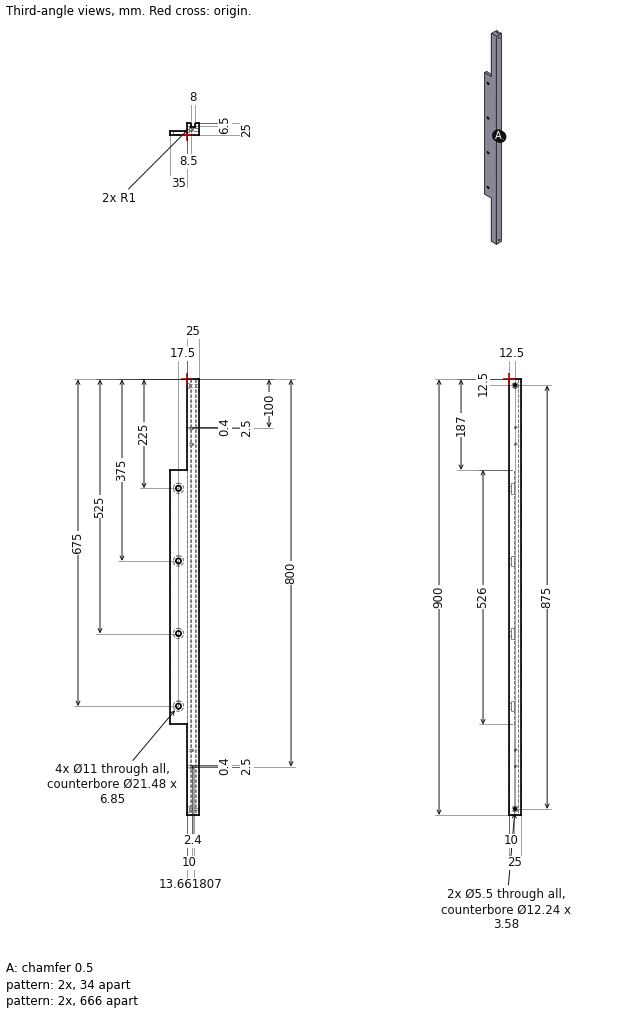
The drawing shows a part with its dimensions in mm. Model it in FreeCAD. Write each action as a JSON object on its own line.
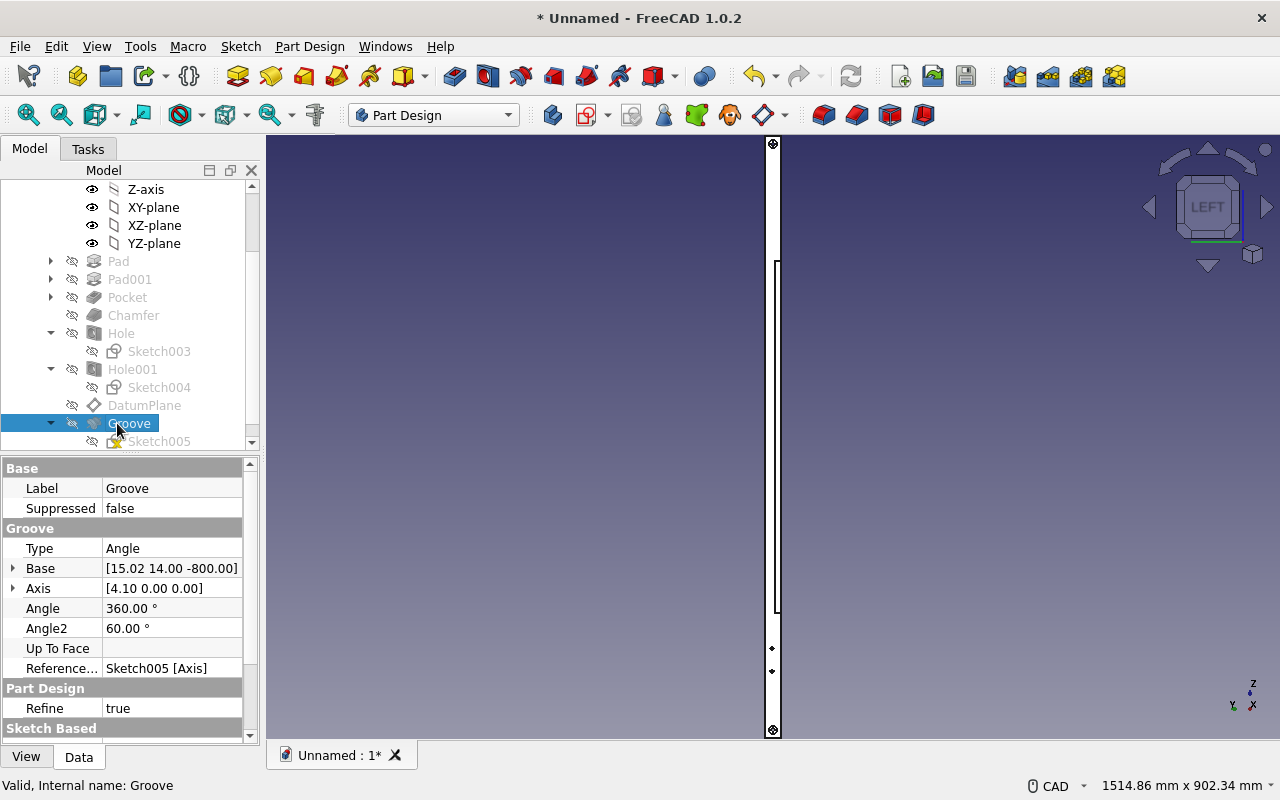
{"action": "left_click", "coordinate": [1048, 76]}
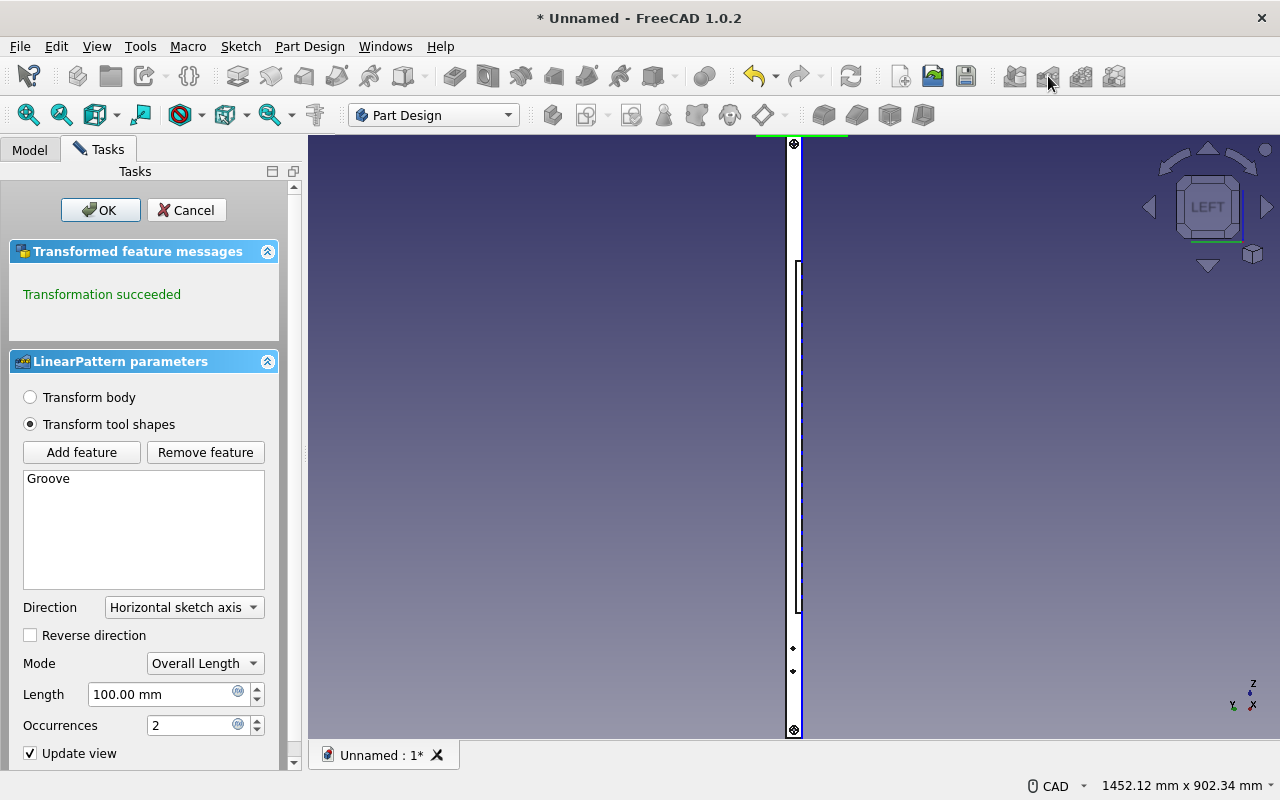
{"action": "left_click", "coordinate": [185, 608]}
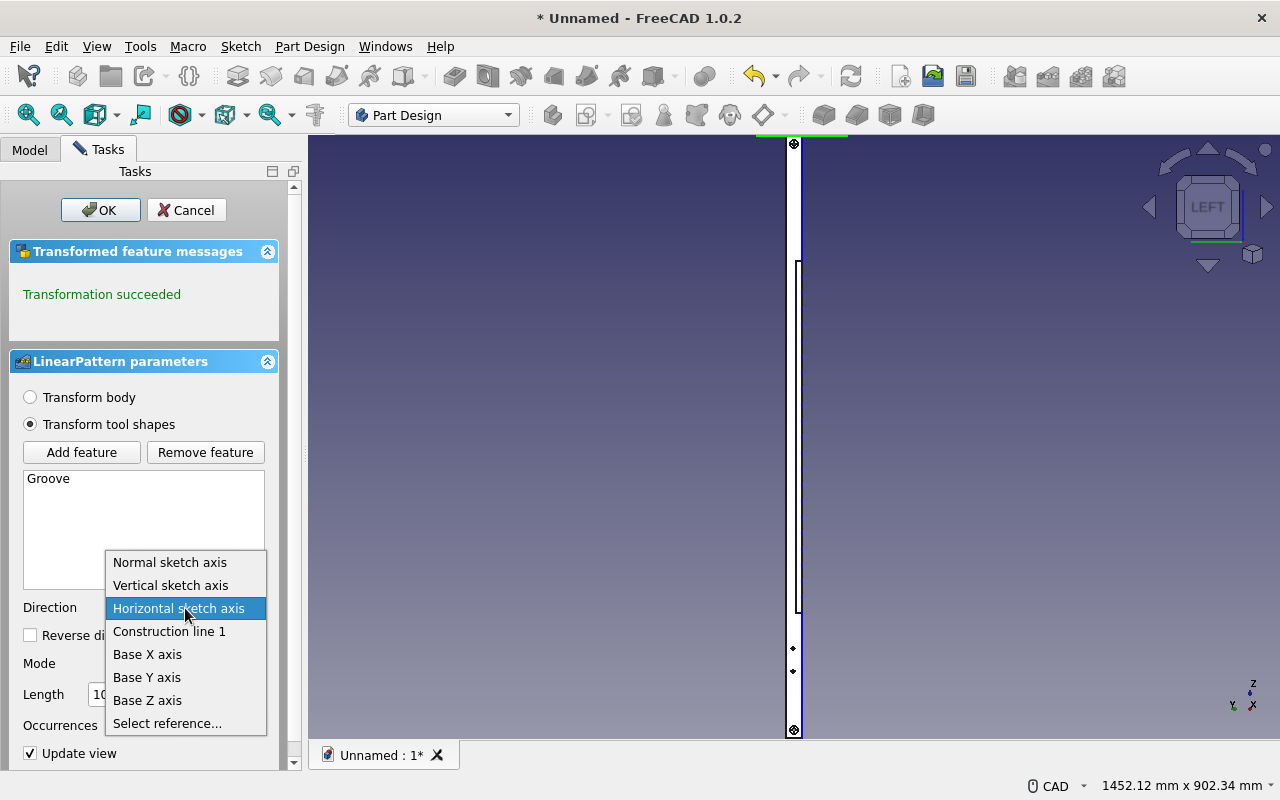
{"action": "left_click", "coordinate": [184, 700]}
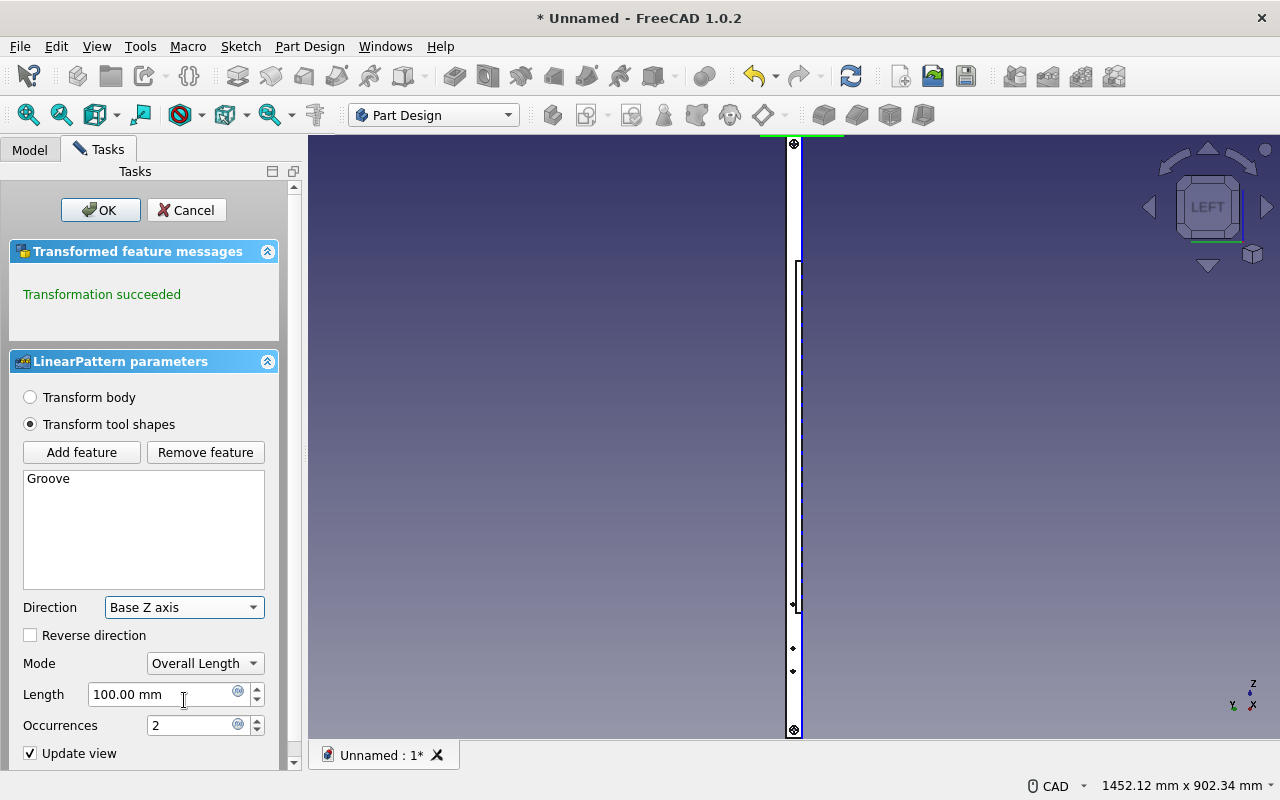
{"action": "left_click", "coordinate": [206, 664]}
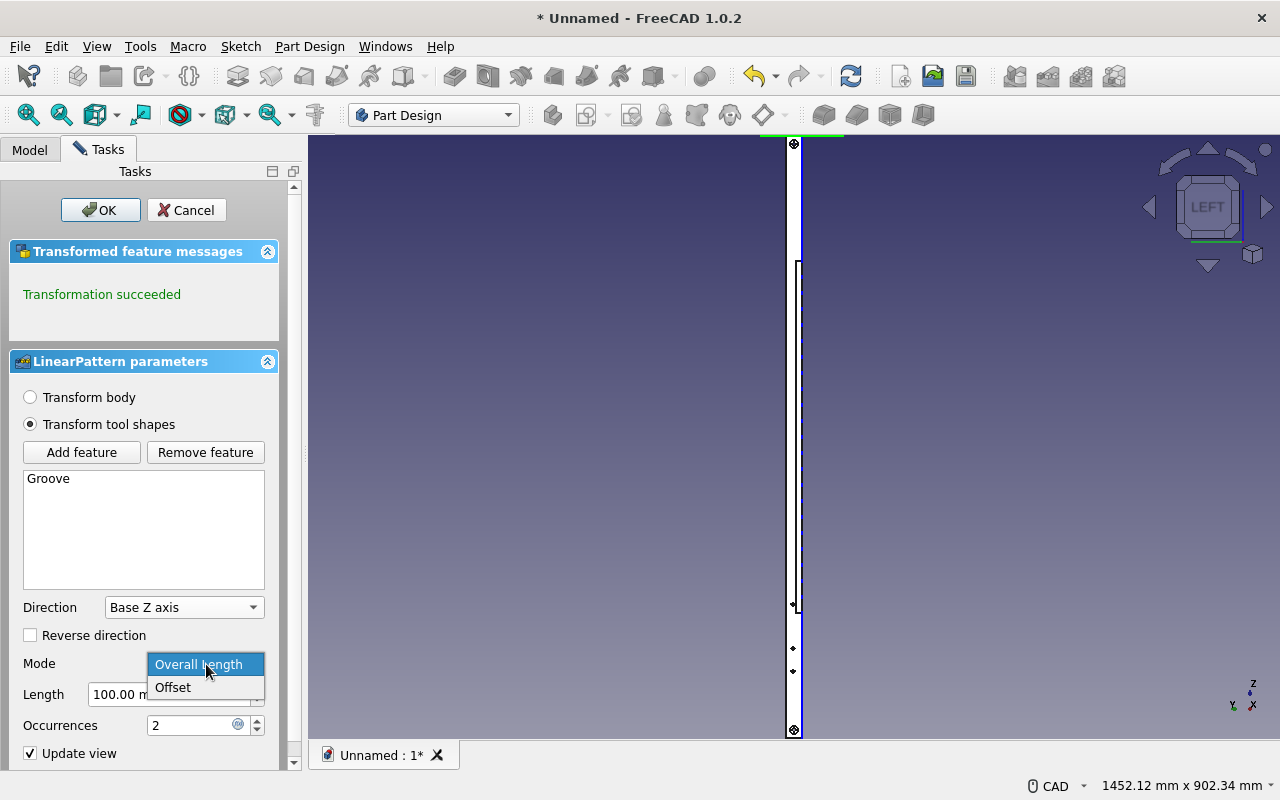
{"action": "left_click", "coordinate": [204, 688]}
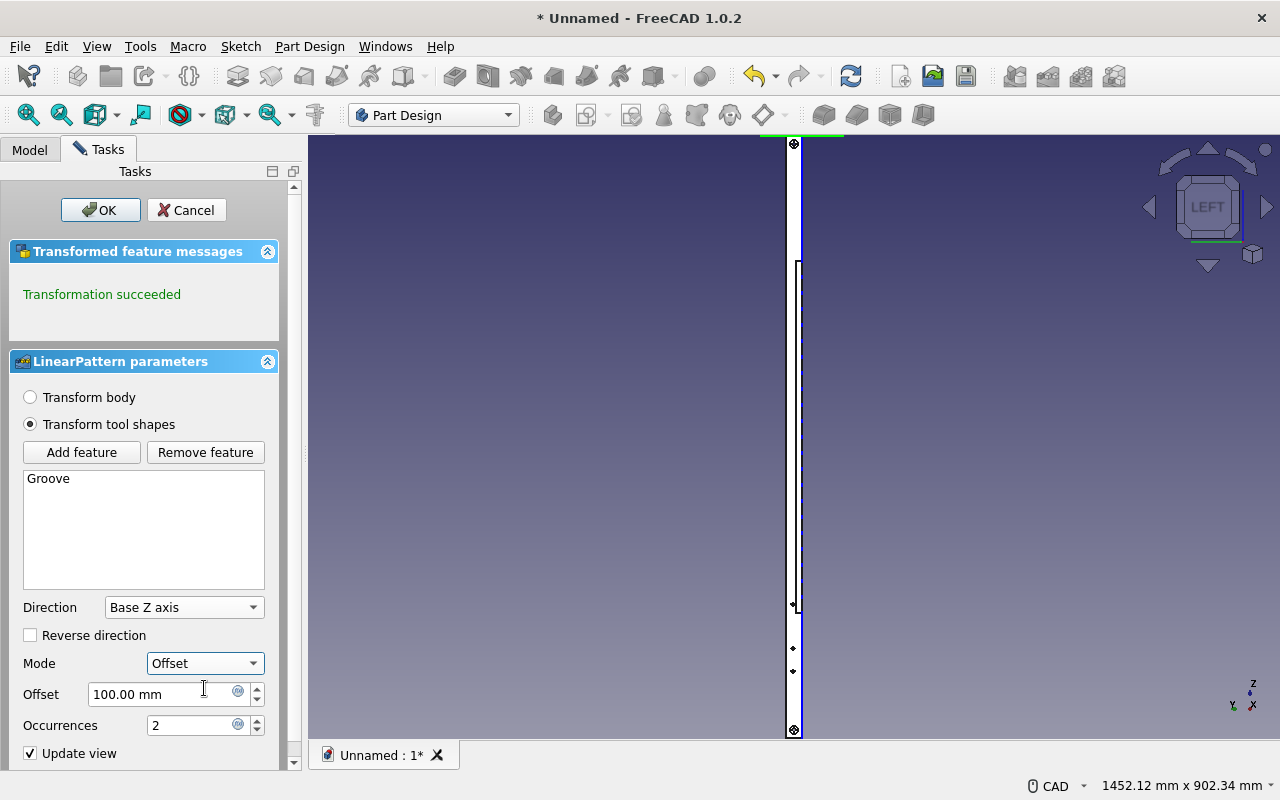
{"action": "triple_click", "coordinate": [170, 694]}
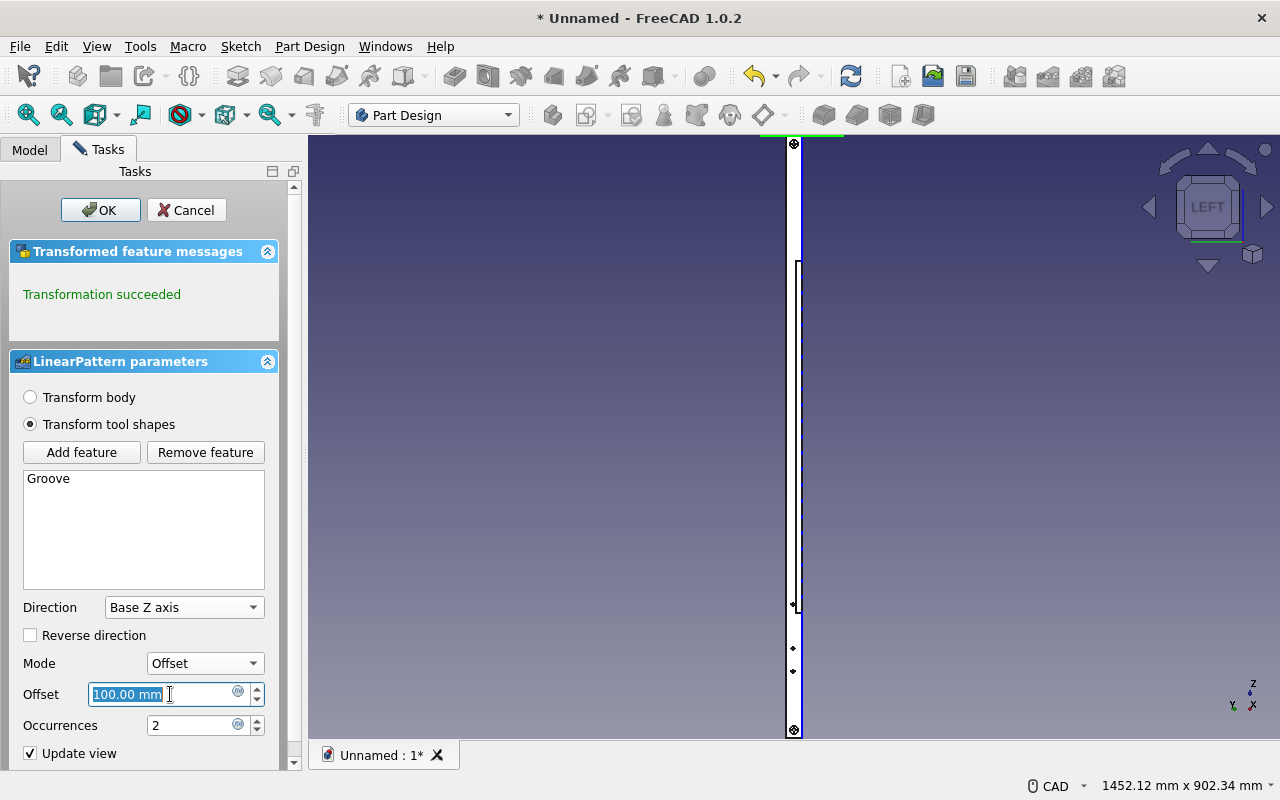
{"action": "type", "text": "666"}
{"action": "key", "text": "Tab"}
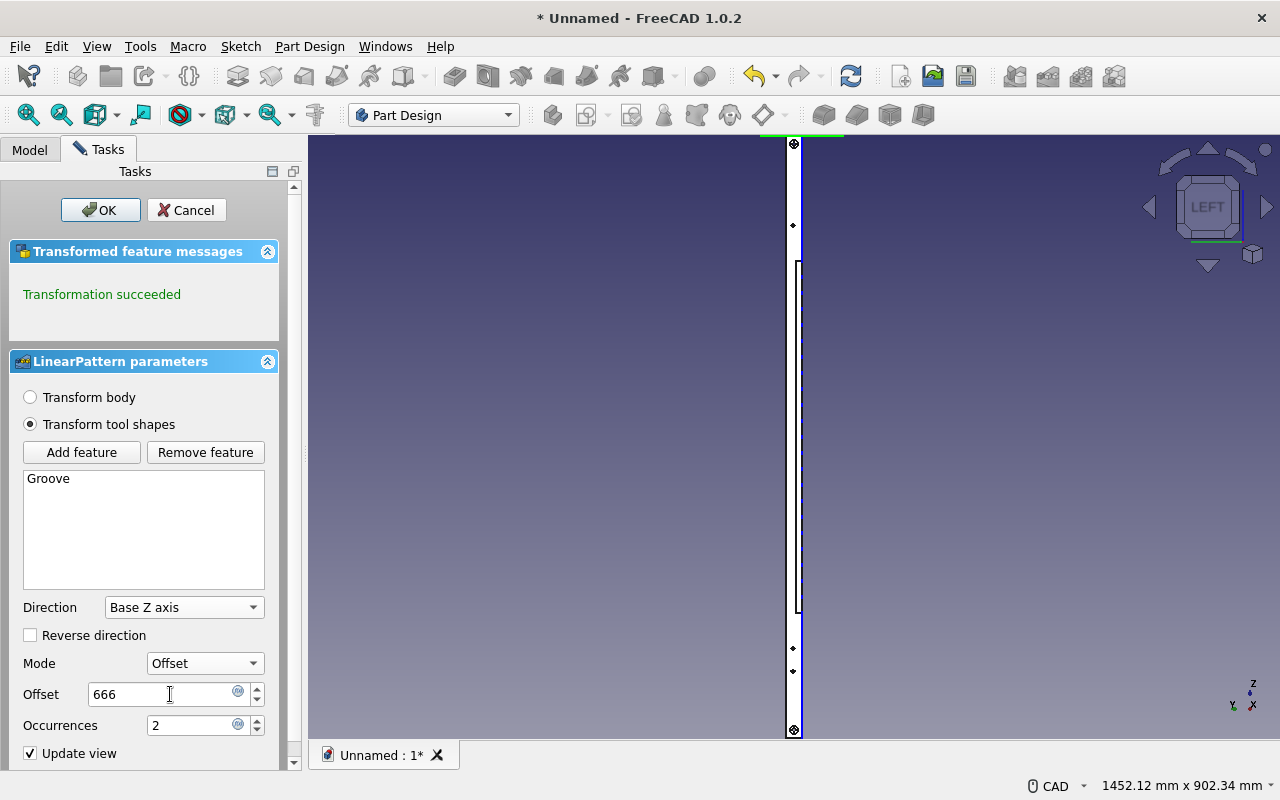
{"action": "triple_click", "coordinate": [199, 726]}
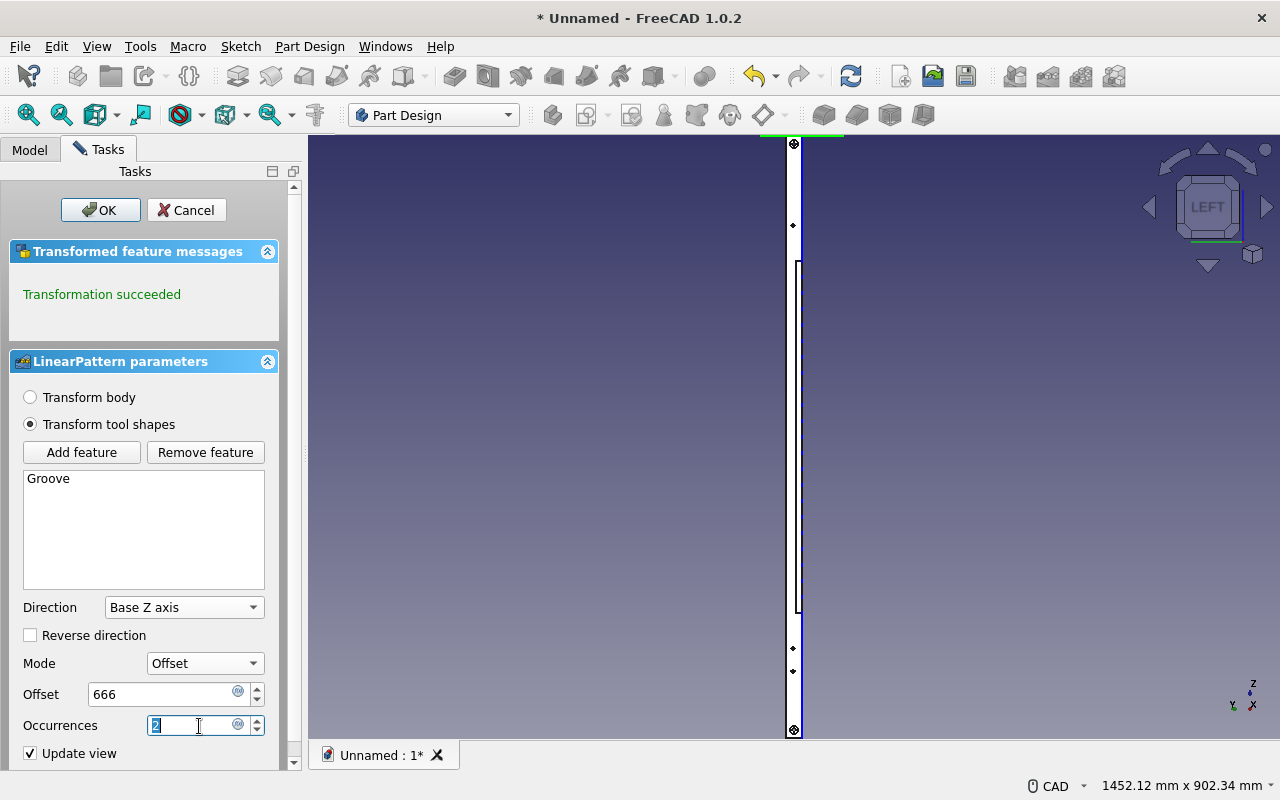
{"action": "type", "text": "2"}
{"action": "key", "text": "Tab"}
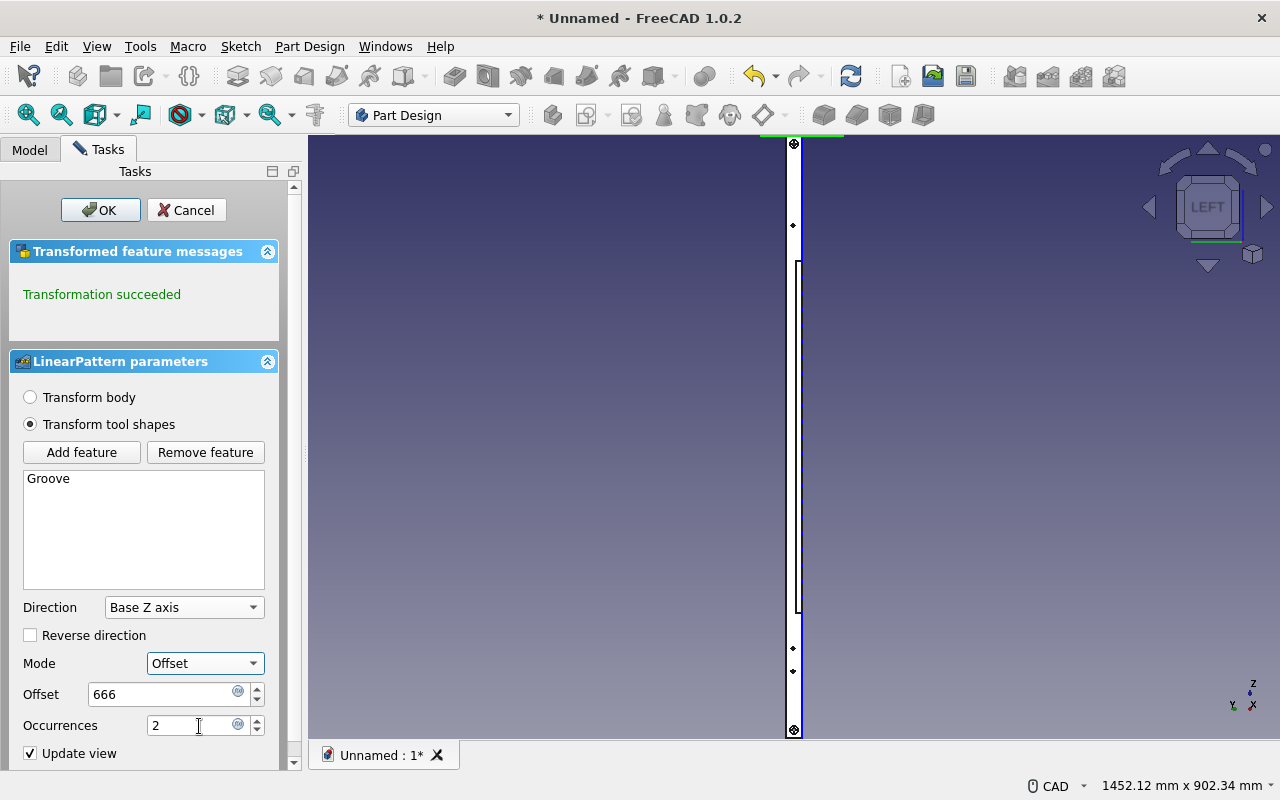
{"action": "left_click", "coordinate": [101, 210]}